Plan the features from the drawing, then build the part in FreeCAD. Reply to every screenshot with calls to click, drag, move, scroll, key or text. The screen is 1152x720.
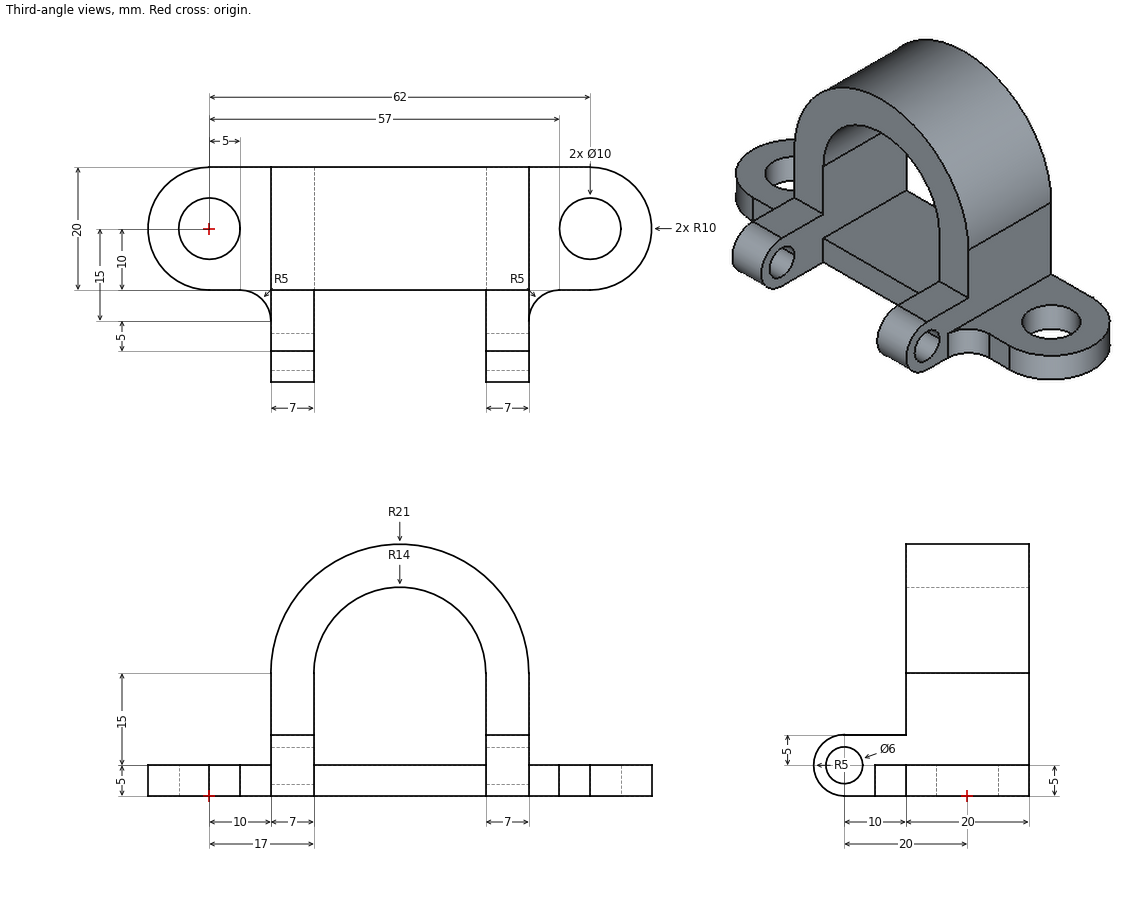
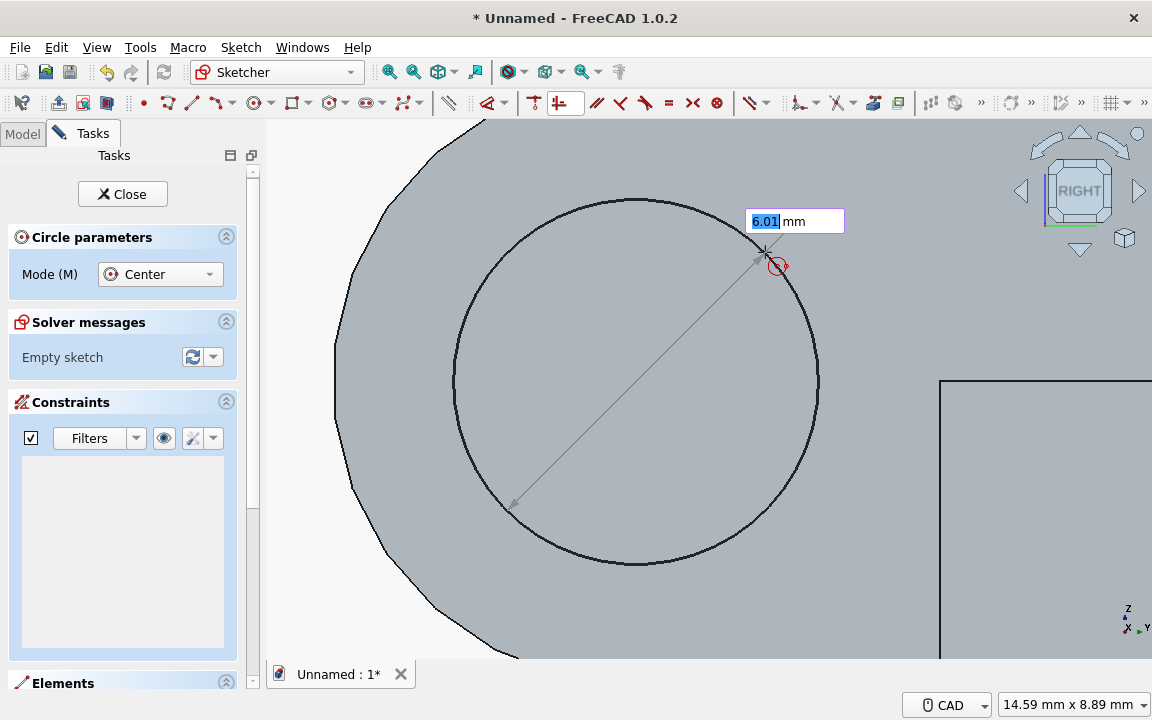
text(6)
key(Return)
key(Escape)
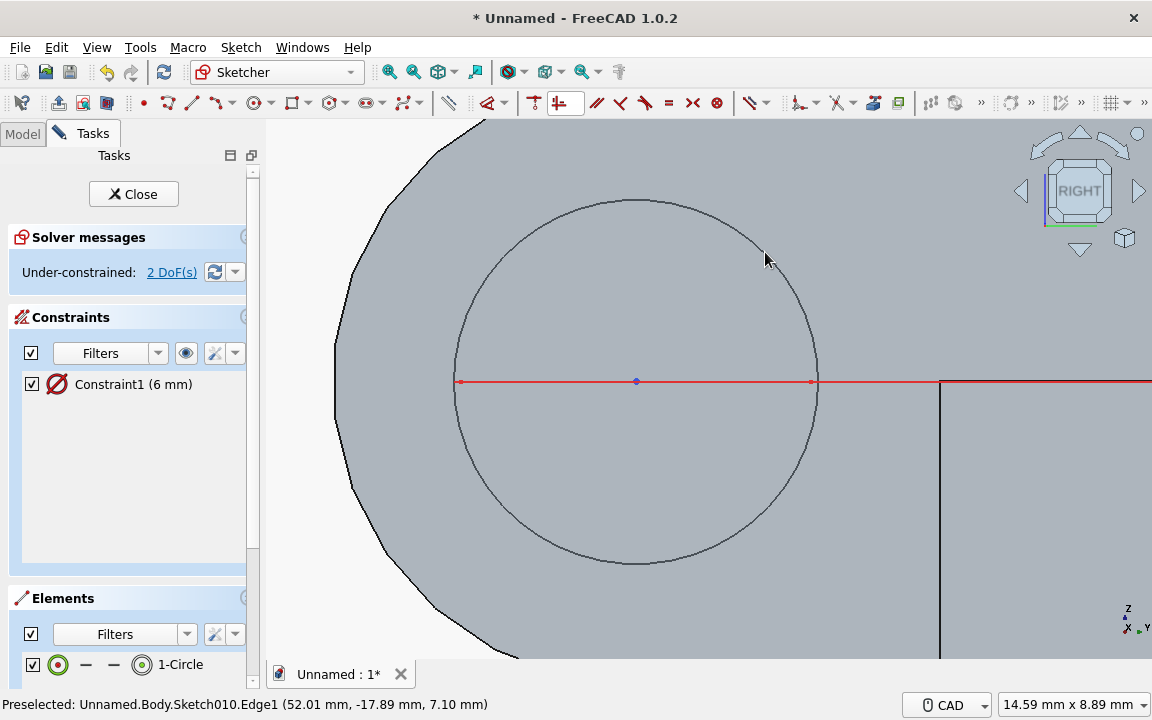
click(488, 104)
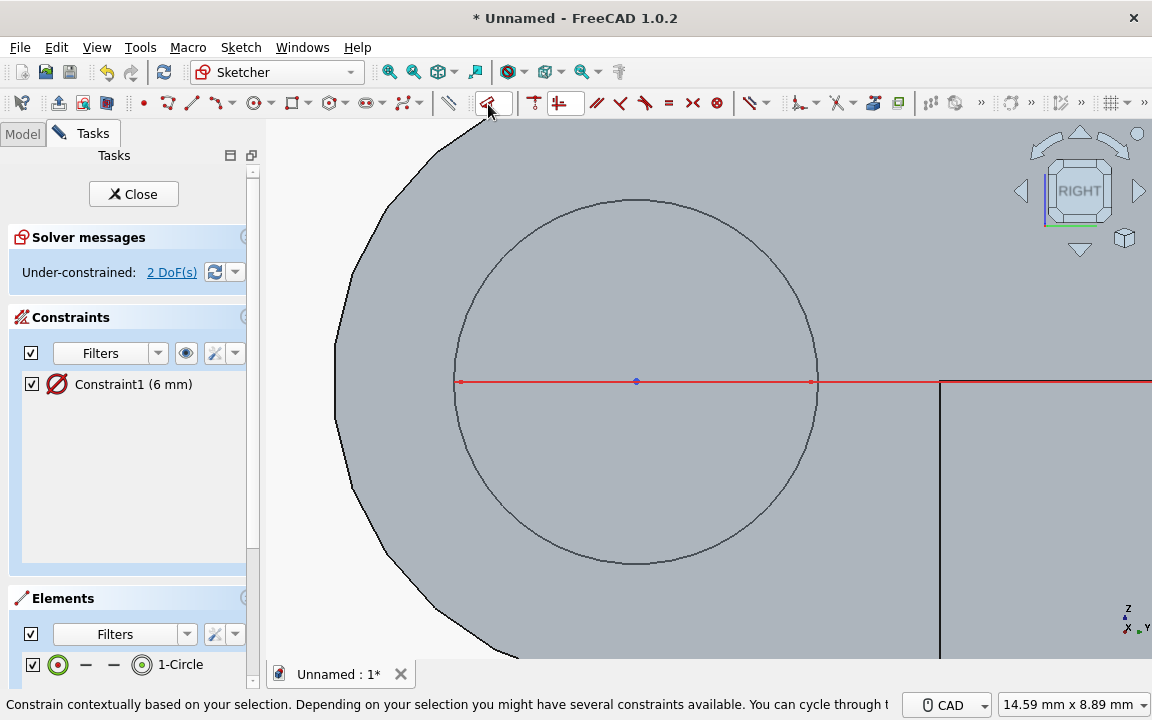
click(636, 382)
click(602, 507)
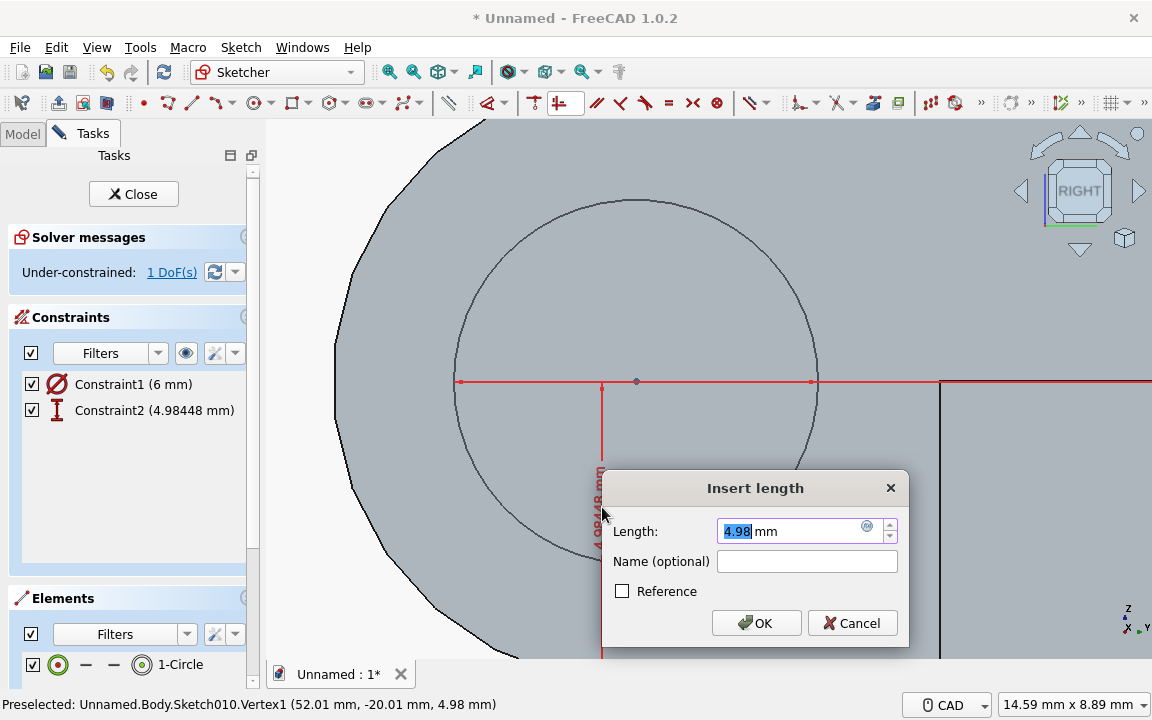
text(5)
key(Return)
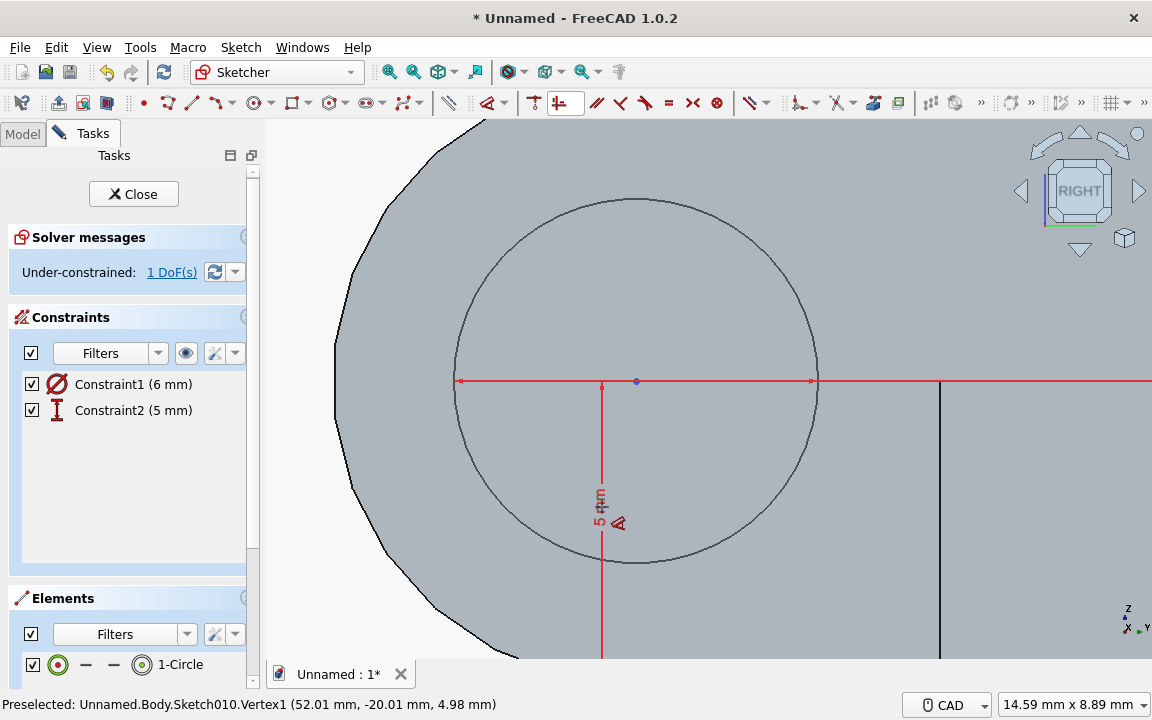
click(636, 381)
click(731, 347)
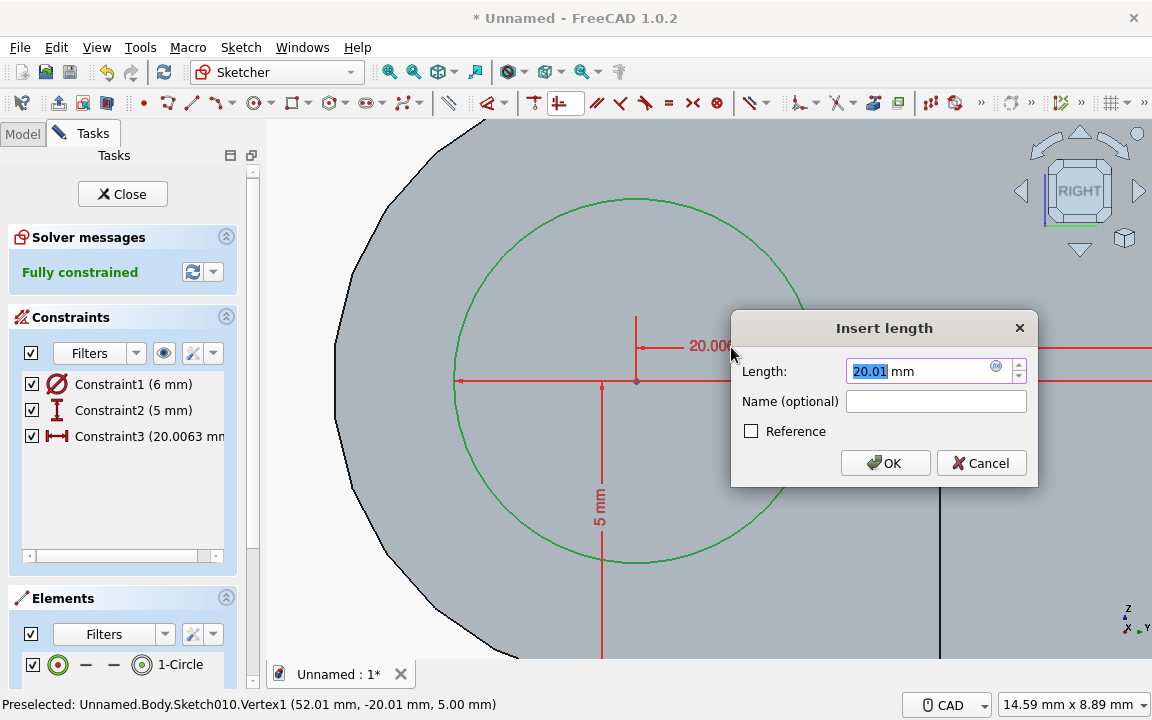
text(20)
key(Return)
key(Escape)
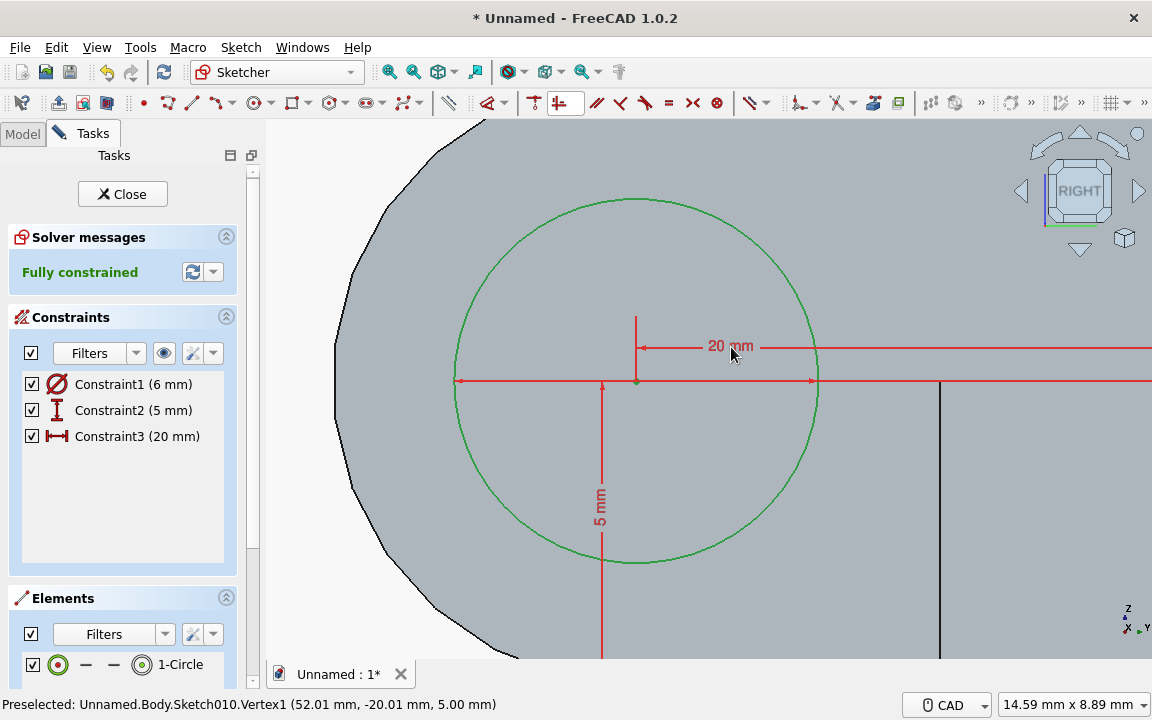
click(123, 194)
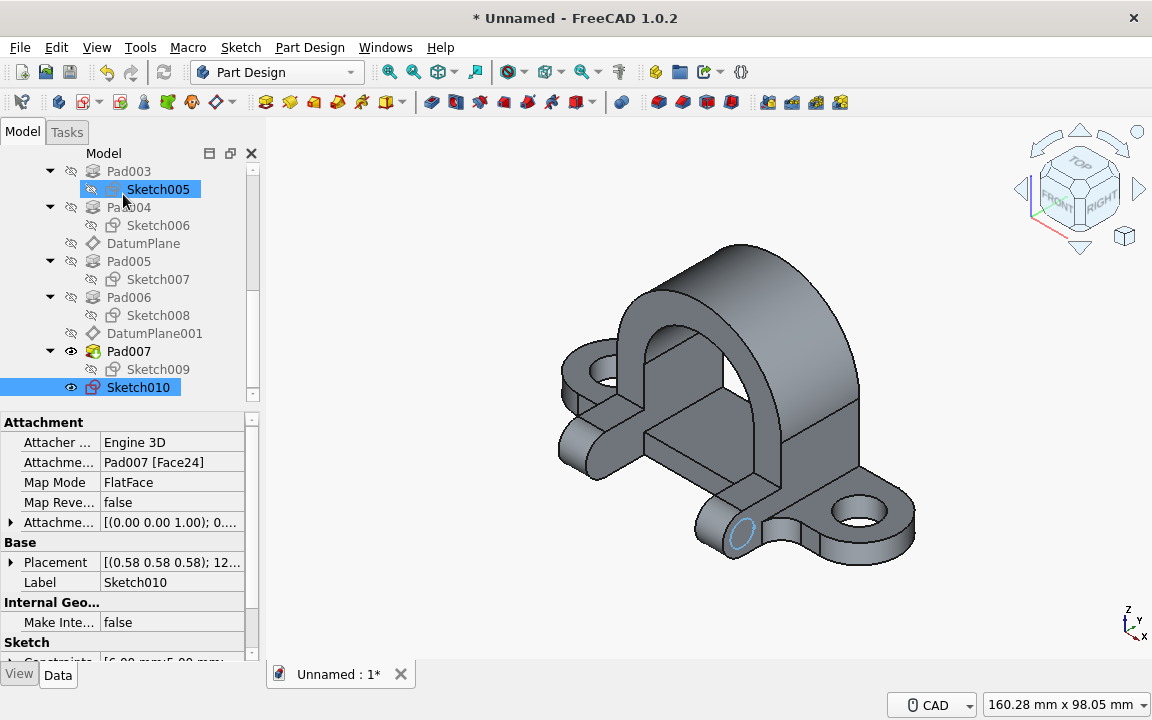
click(432, 102)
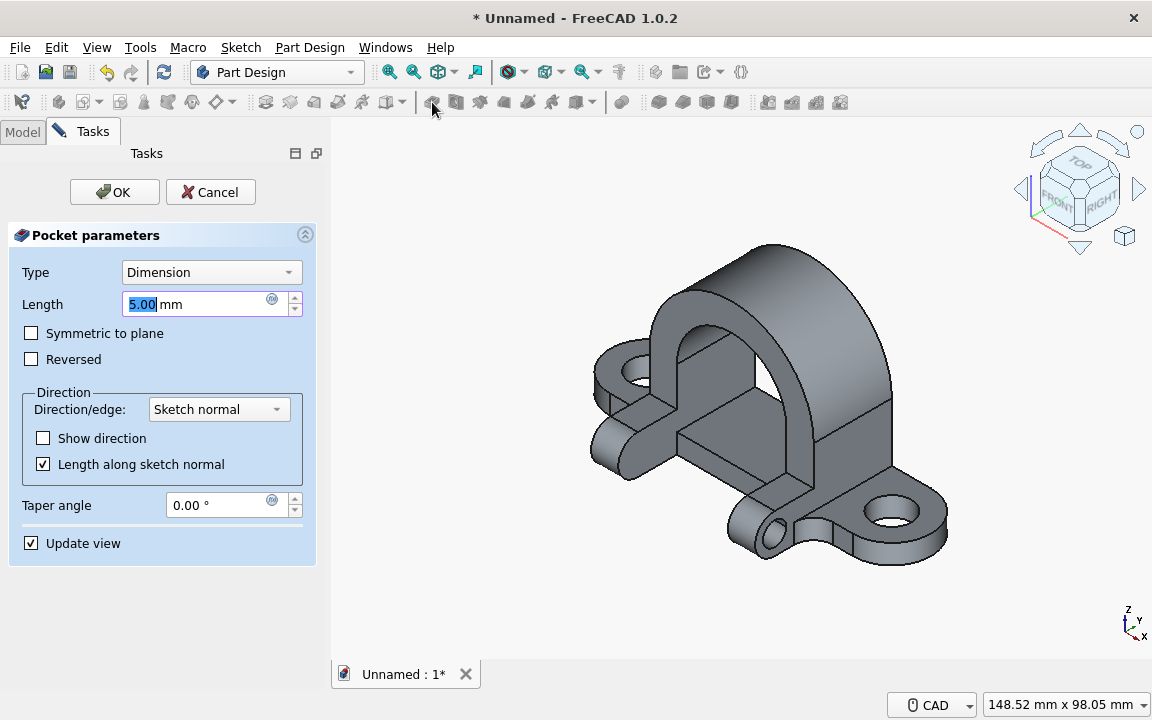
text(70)
key(Tab)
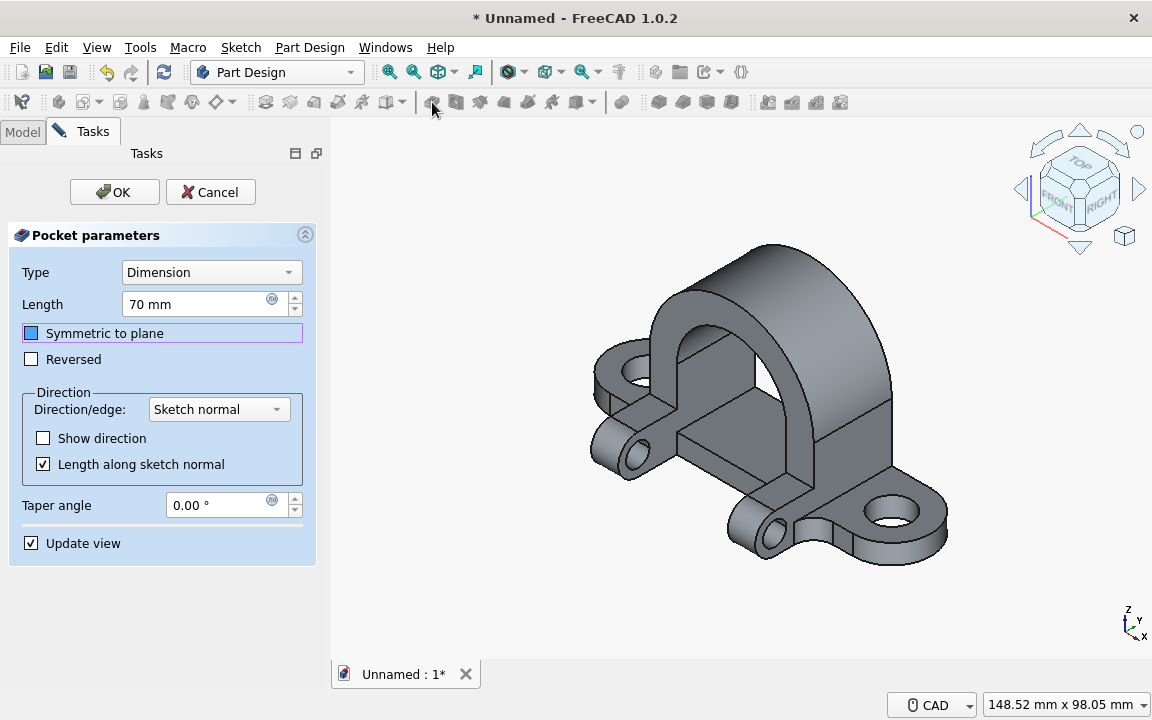
click(115, 192)